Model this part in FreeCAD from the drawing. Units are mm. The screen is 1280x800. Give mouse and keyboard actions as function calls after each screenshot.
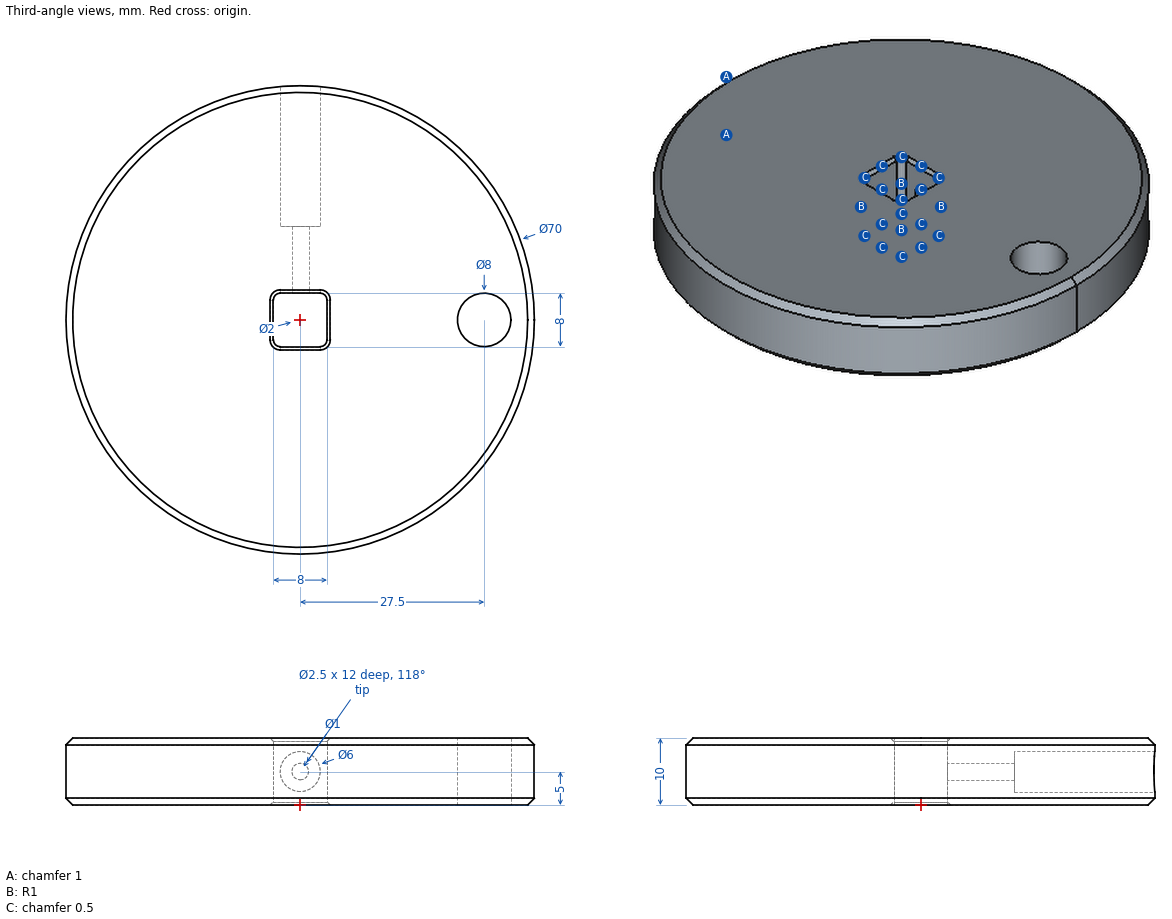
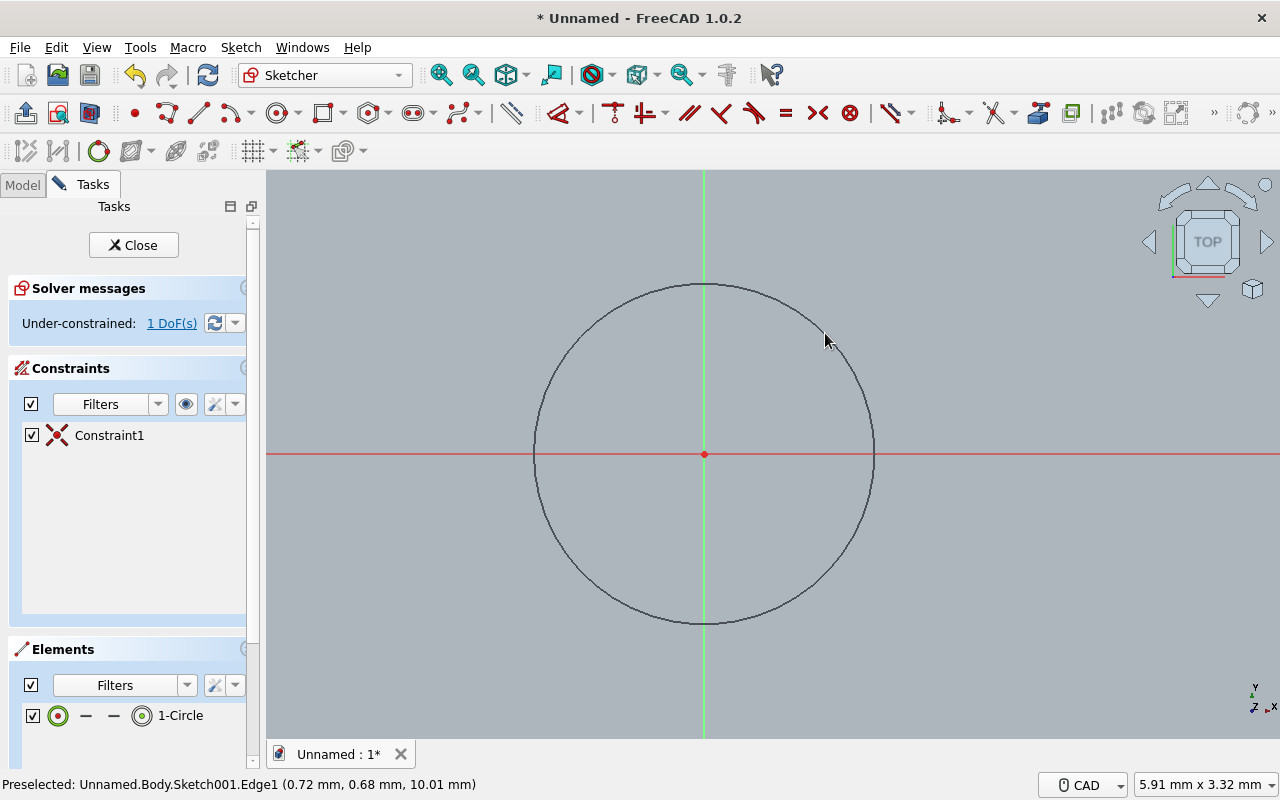
click(558, 114)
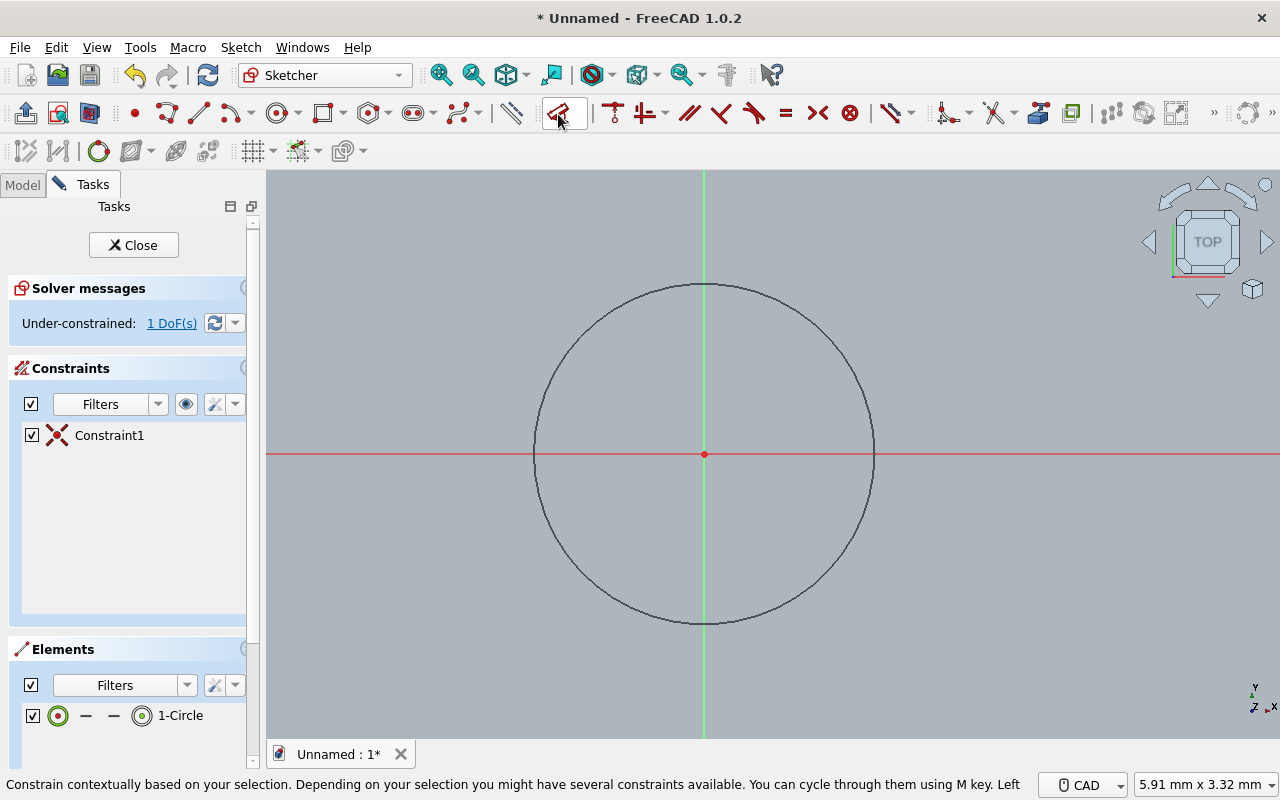
click(824, 333)
click(847, 310)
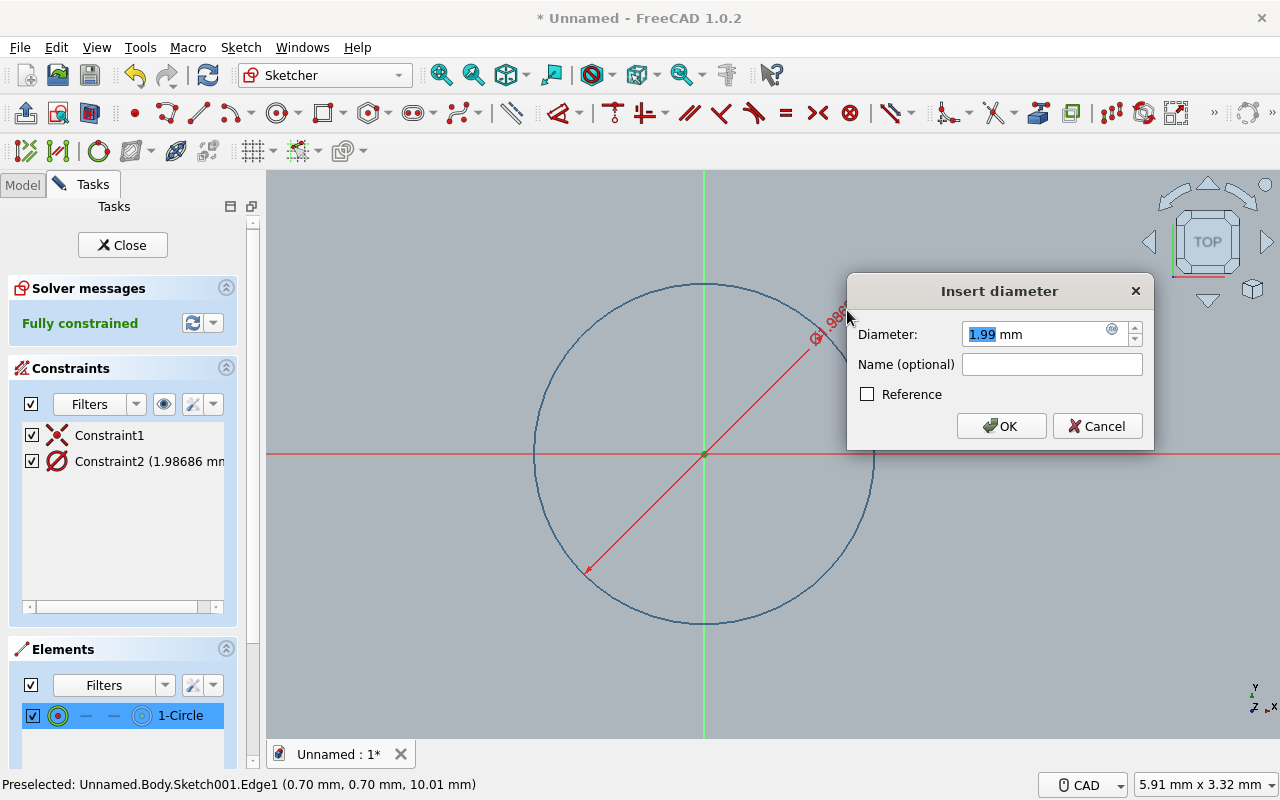
text(2)
key(Return)
key(Escape)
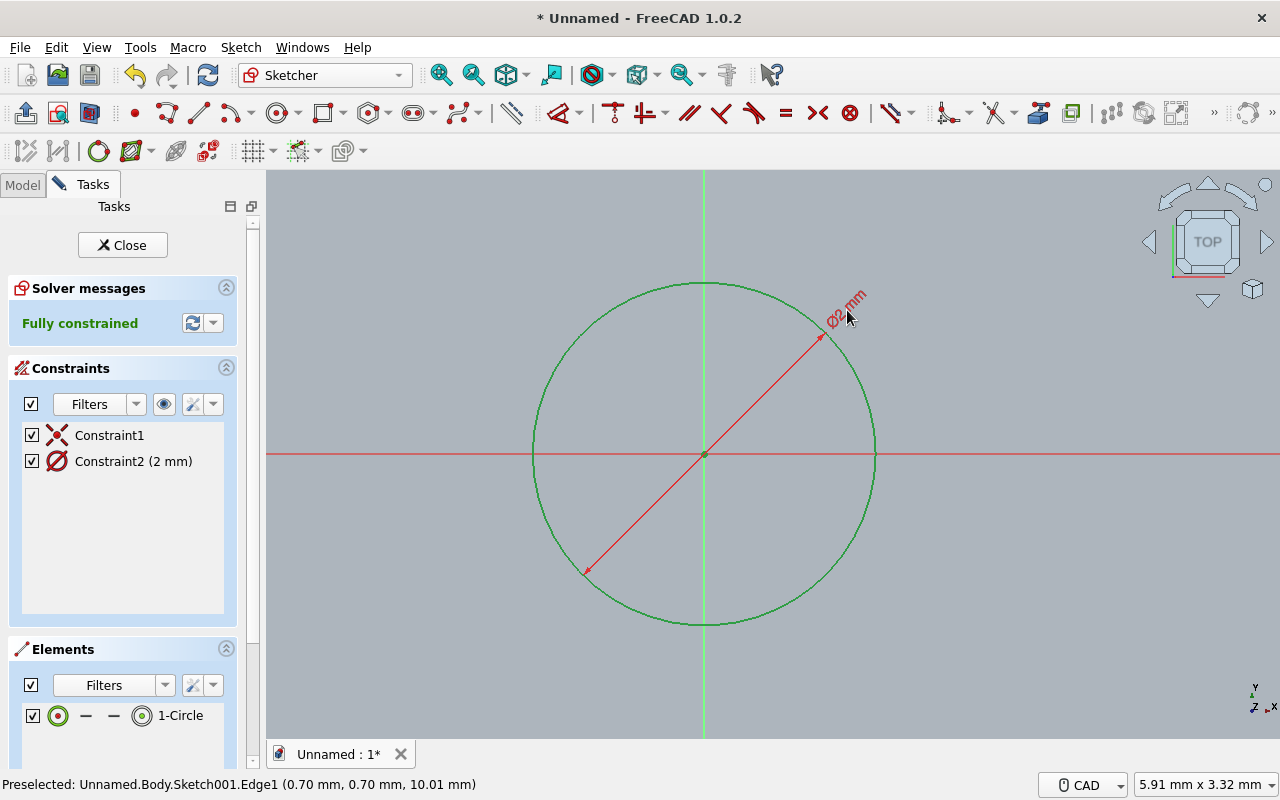
click(123, 245)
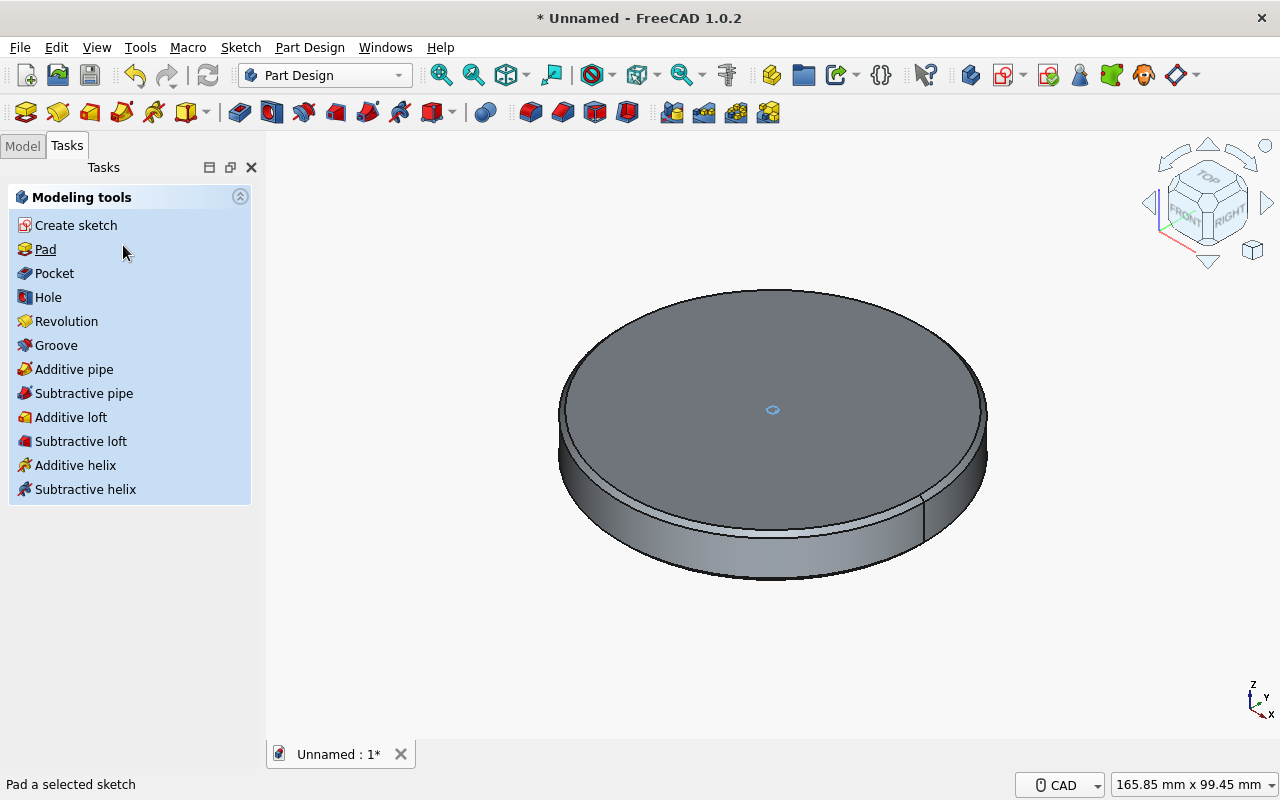
click(240, 112)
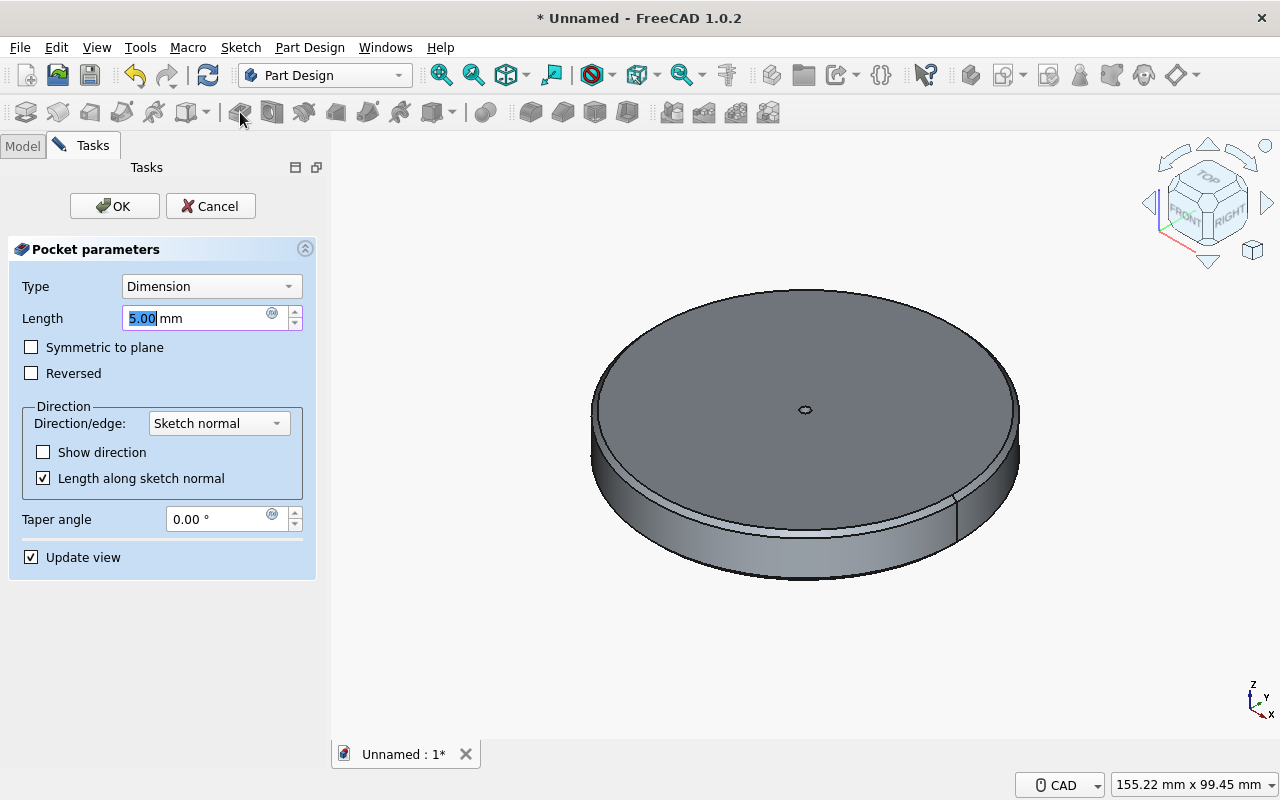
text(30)
key(Tab)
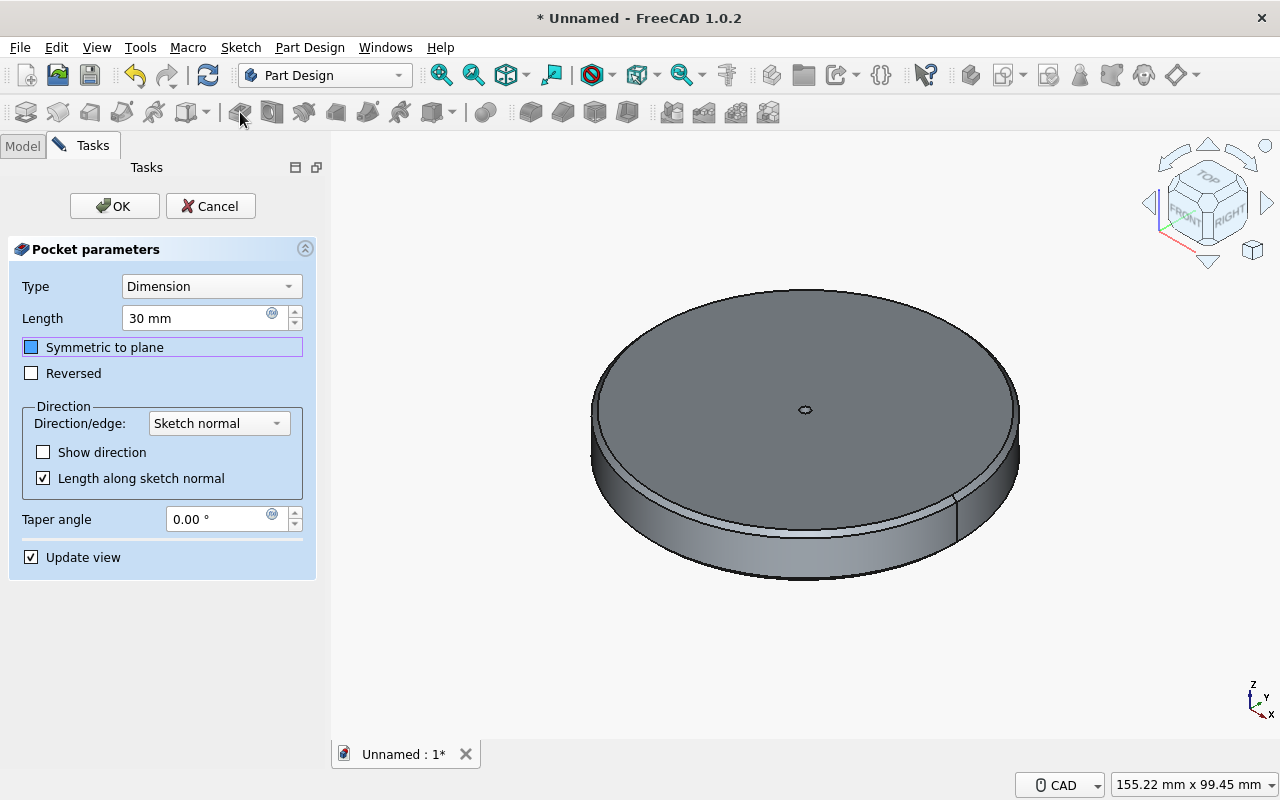
click(115, 206)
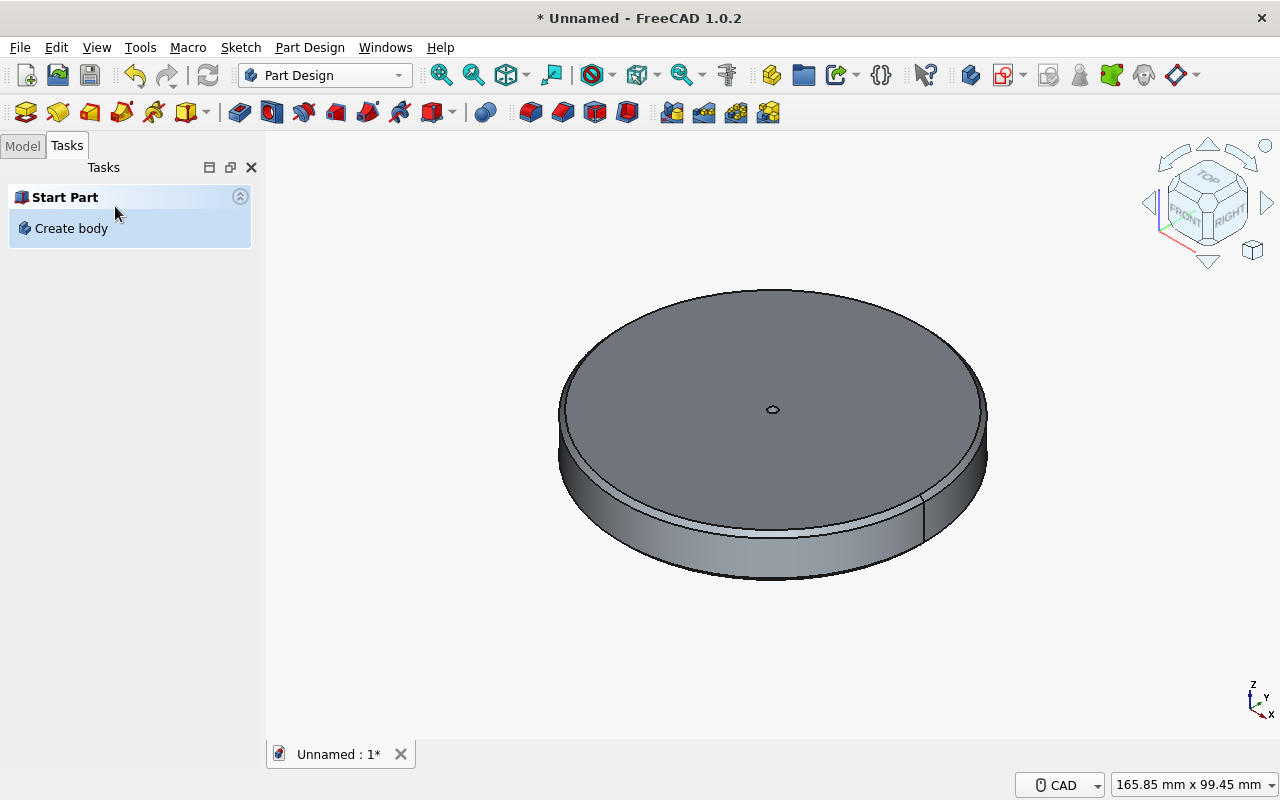
click(689, 457)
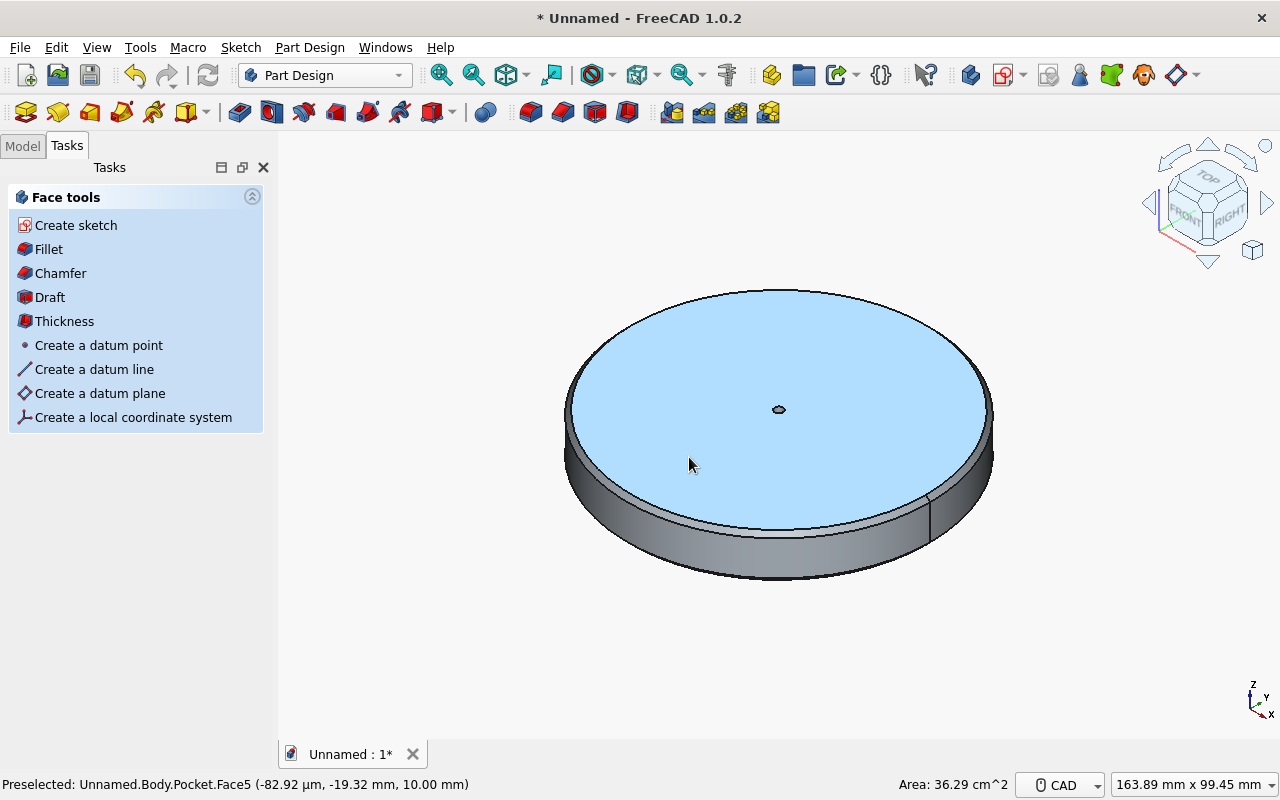
click(1004, 76)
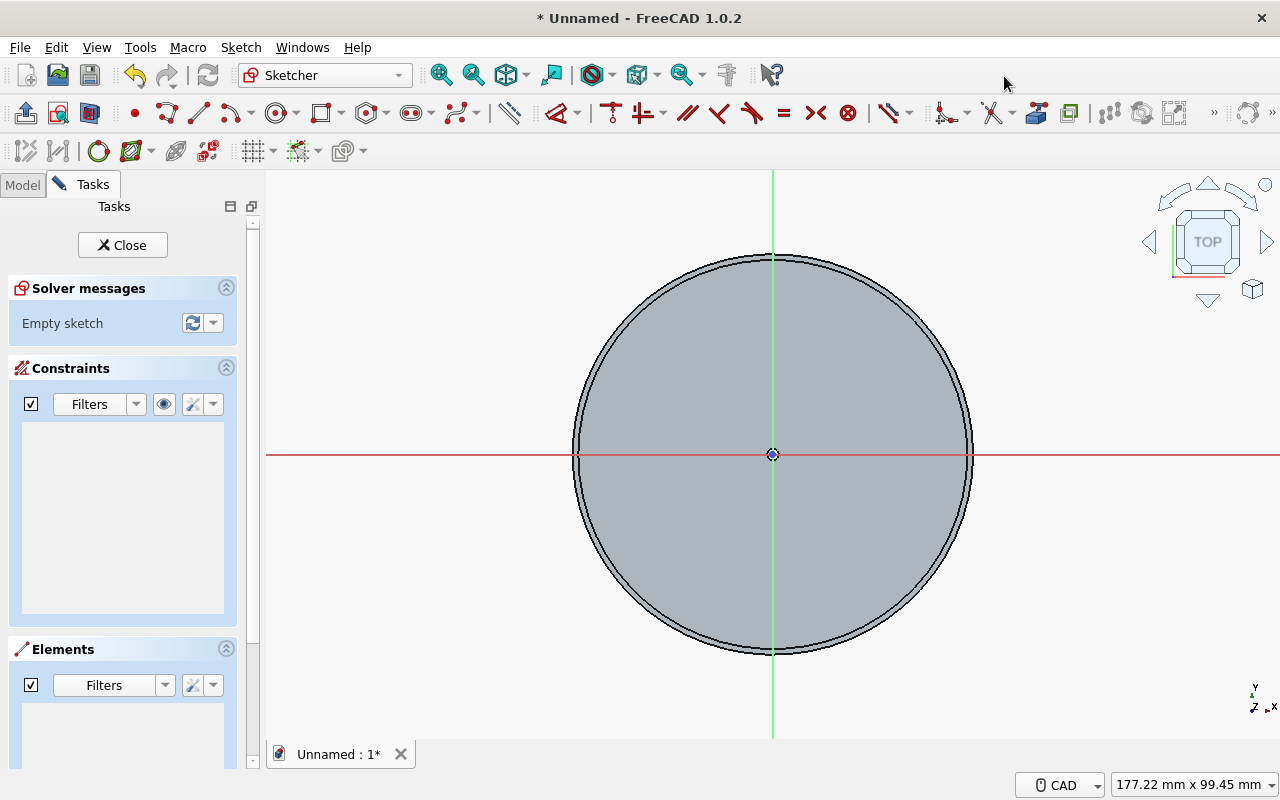
scroll(966, 454, up, 10)